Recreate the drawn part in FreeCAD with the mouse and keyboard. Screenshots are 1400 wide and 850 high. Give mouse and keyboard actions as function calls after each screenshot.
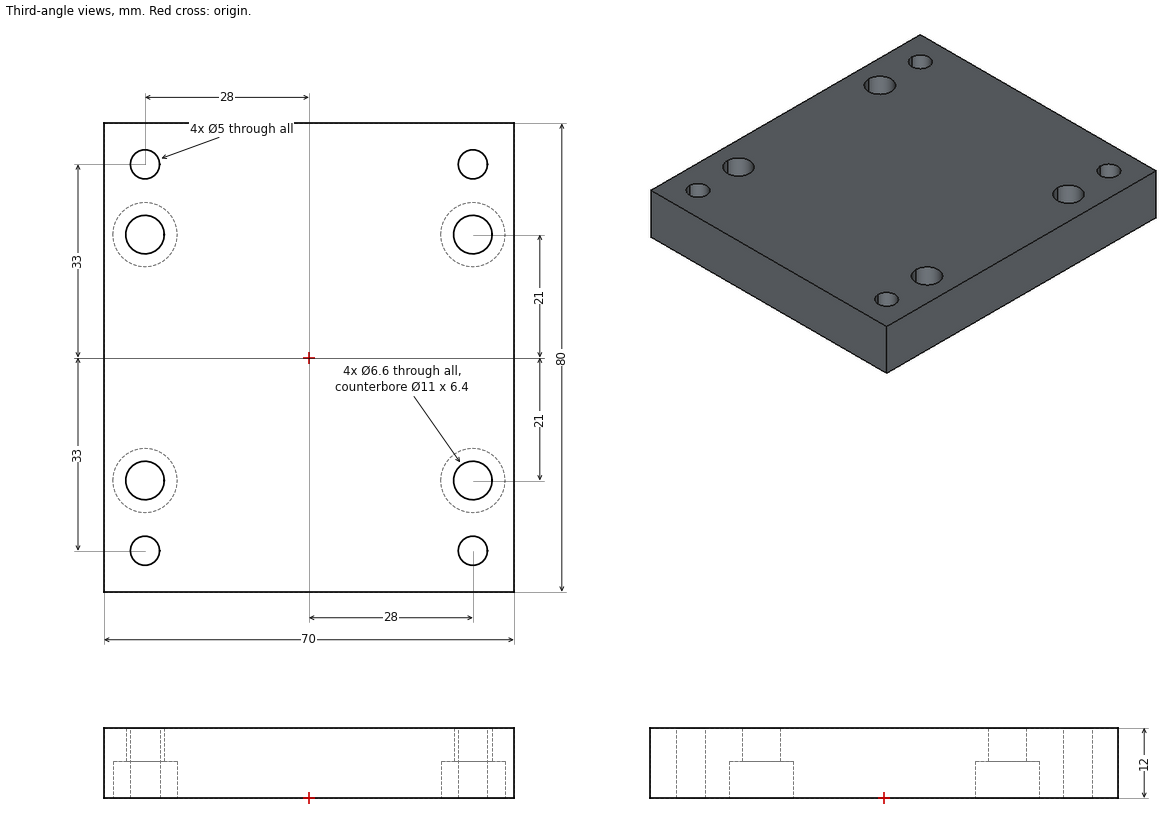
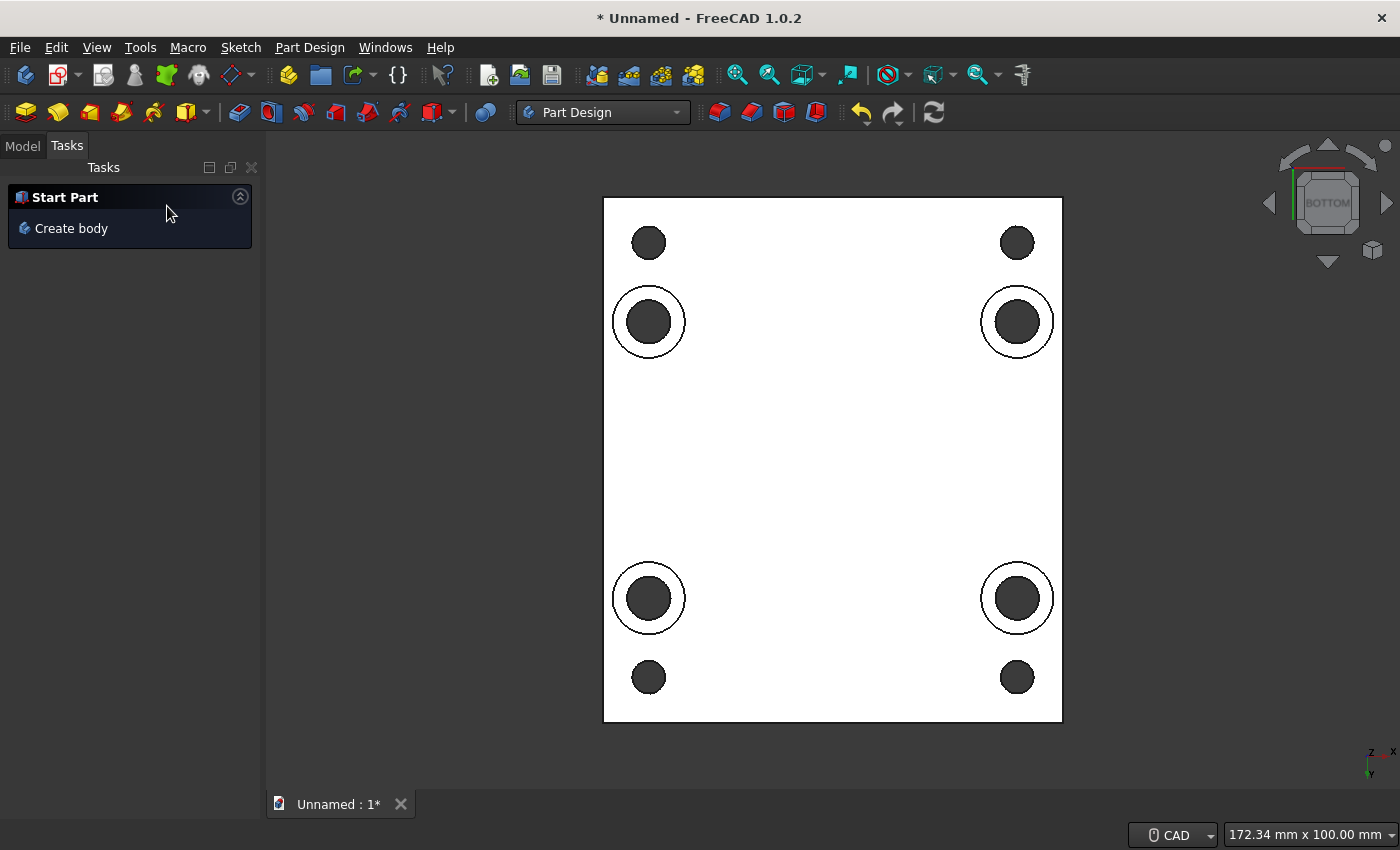
key(0)